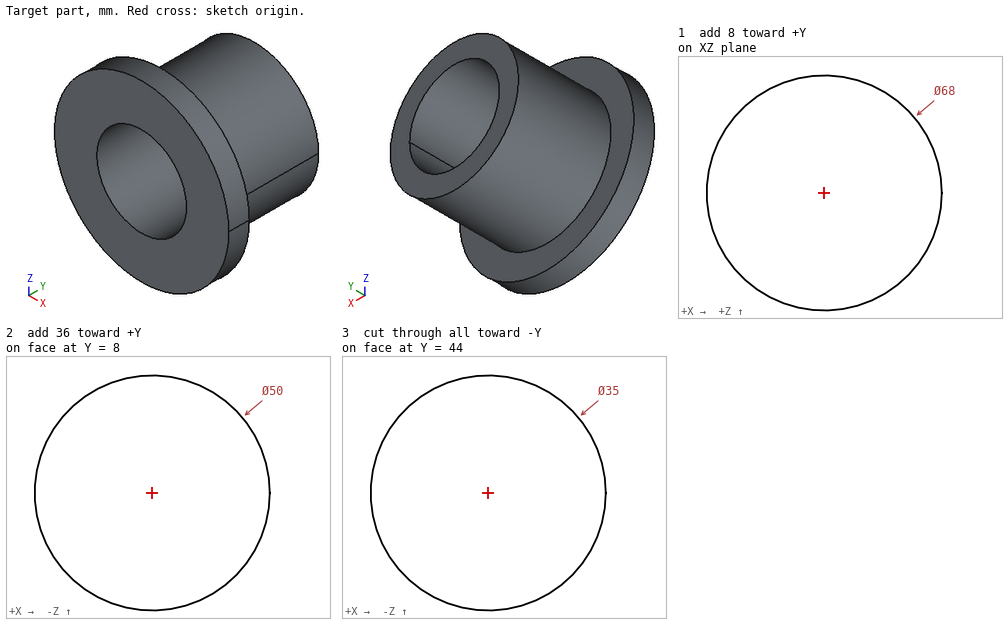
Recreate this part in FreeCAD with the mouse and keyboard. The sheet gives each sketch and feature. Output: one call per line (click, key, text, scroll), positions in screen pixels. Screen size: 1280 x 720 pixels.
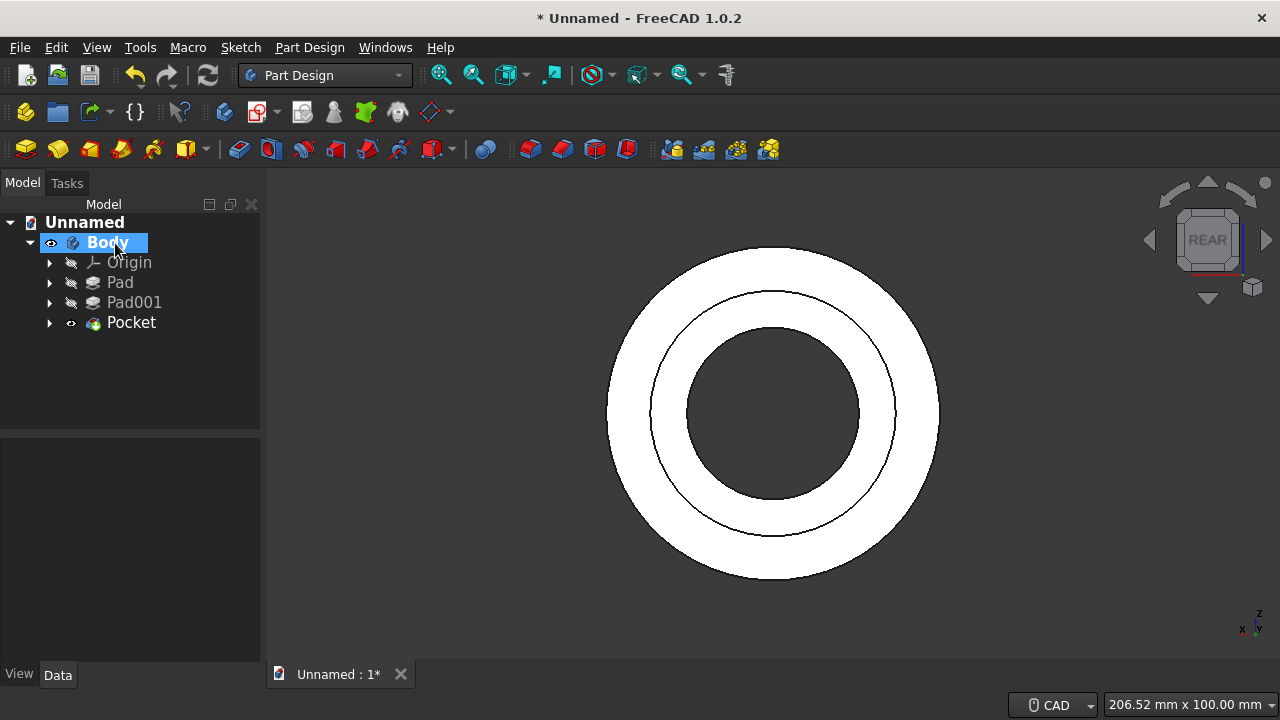
key(0)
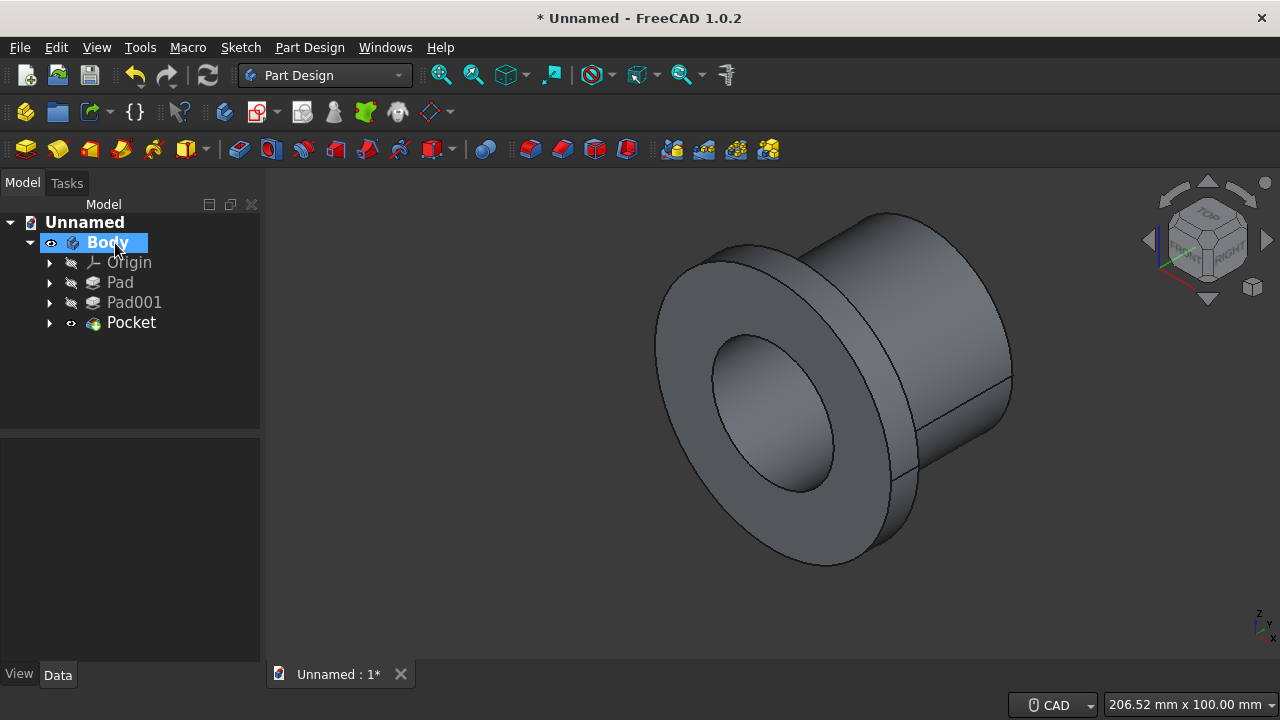
click(442, 76)